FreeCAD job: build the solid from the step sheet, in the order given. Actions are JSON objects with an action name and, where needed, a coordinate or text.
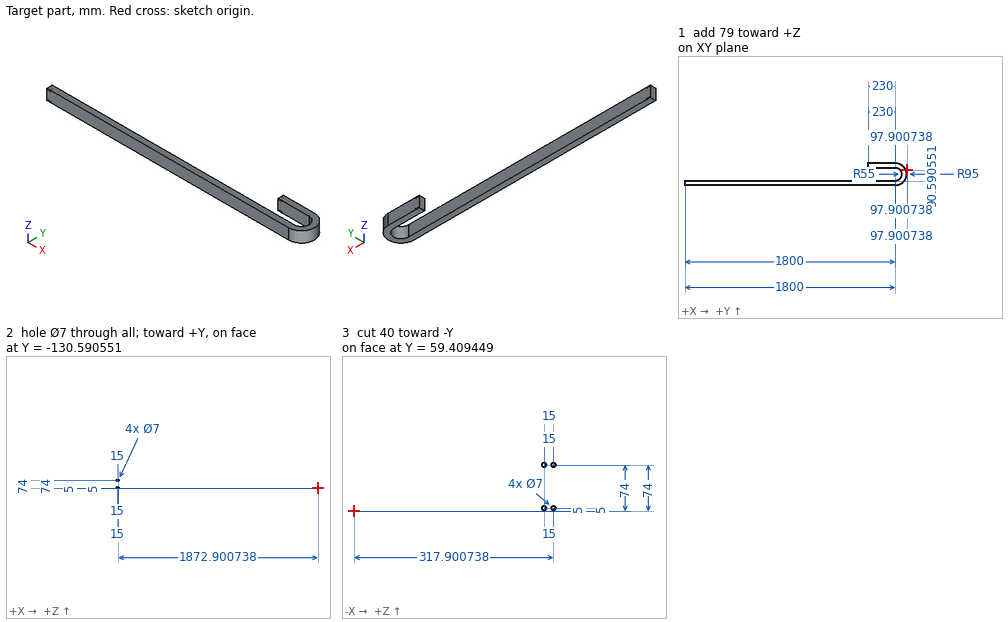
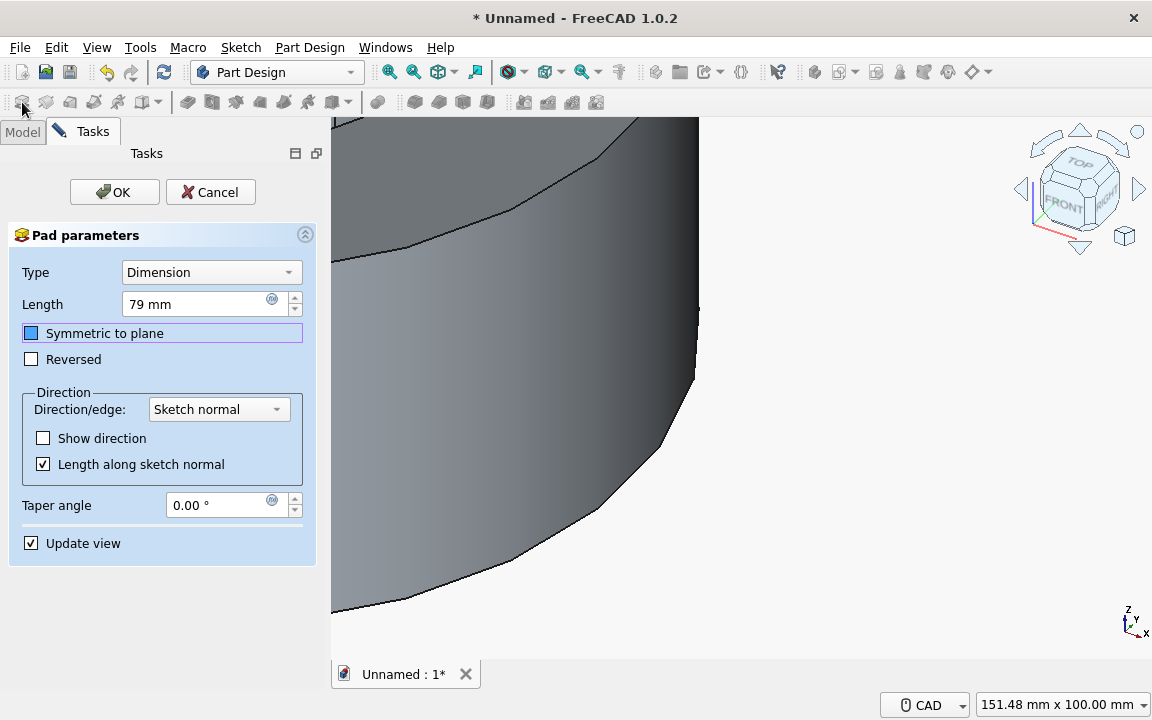
{"action": "left_click", "coordinate": [115, 192]}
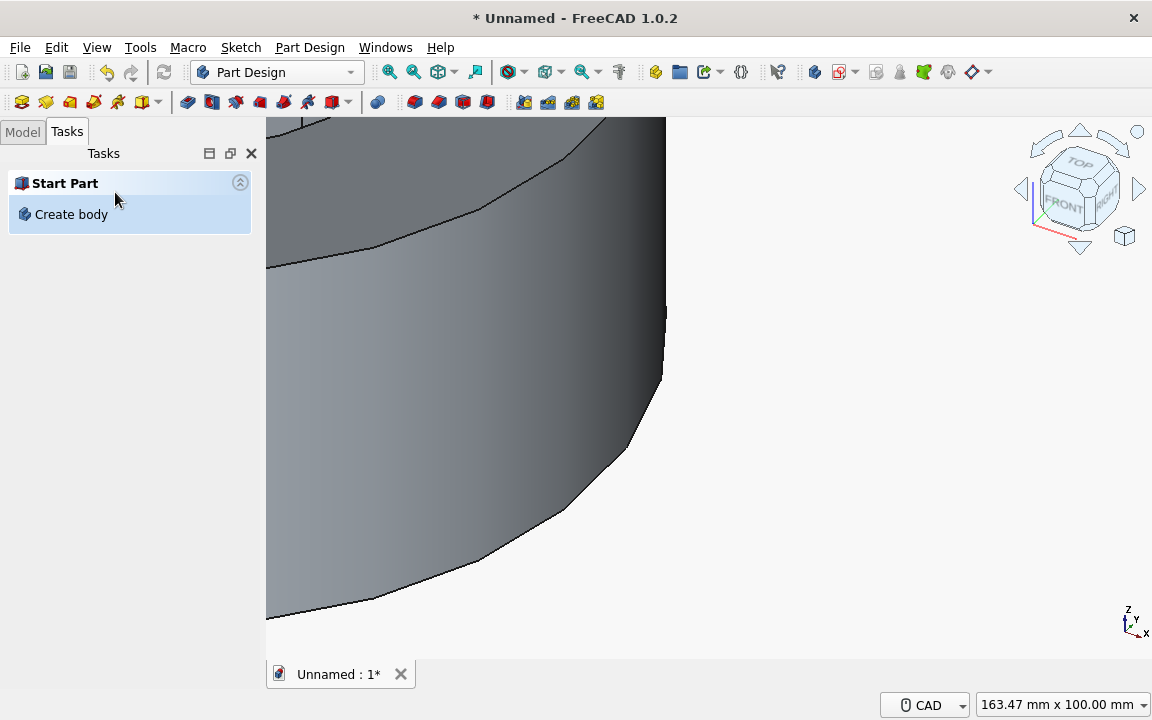
{"action": "left_click", "coordinate": [390, 72]}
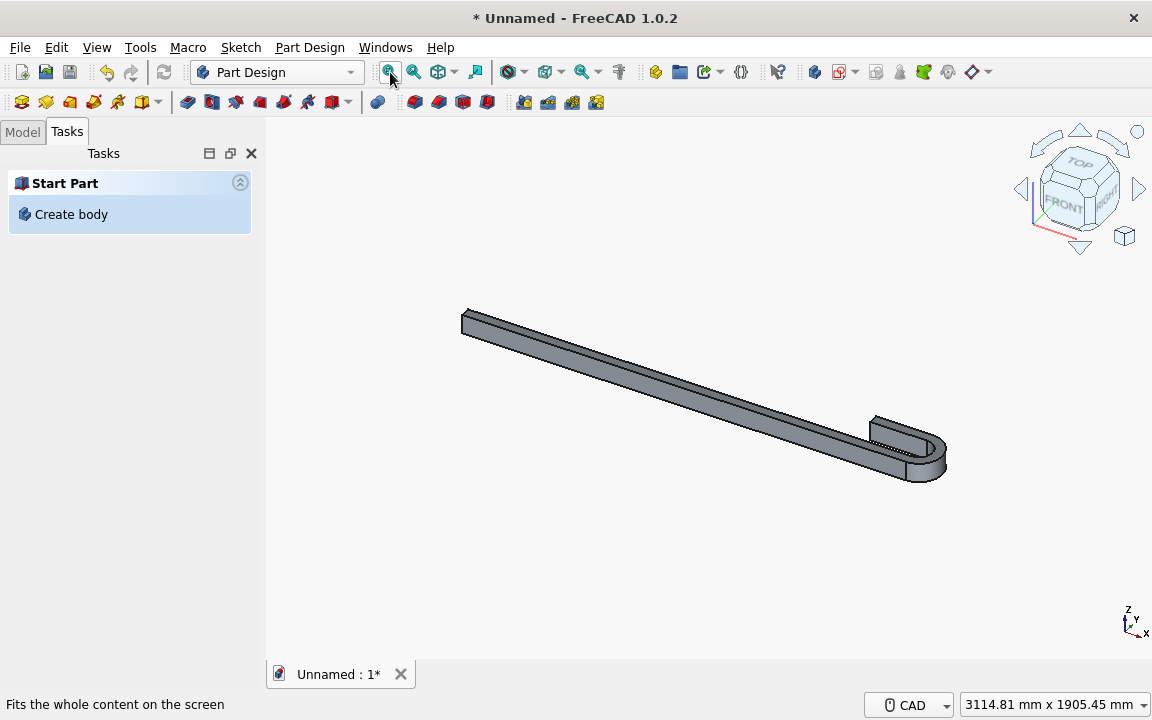
{"action": "left_click", "coordinate": [874, 460]}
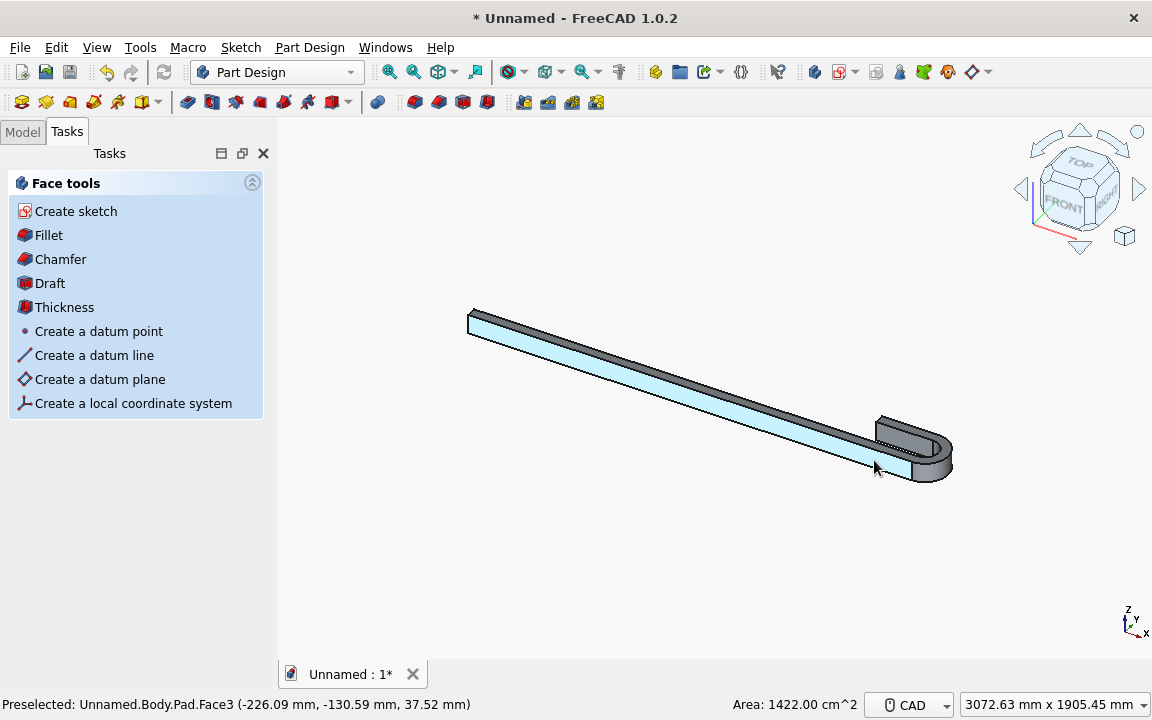
{"action": "left_click", "coordinate": [840, 72]}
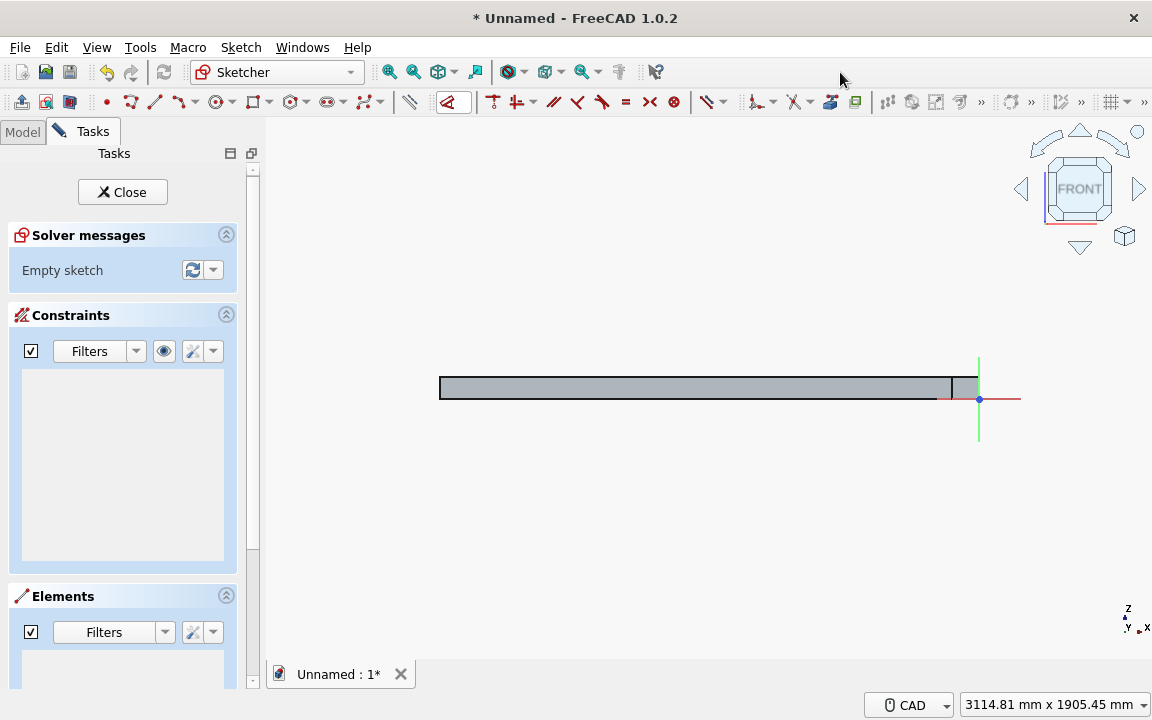
{"action": "scroll", "coordinate": [432, 388], "scroll_direction": "up", "scroll_amount": 14}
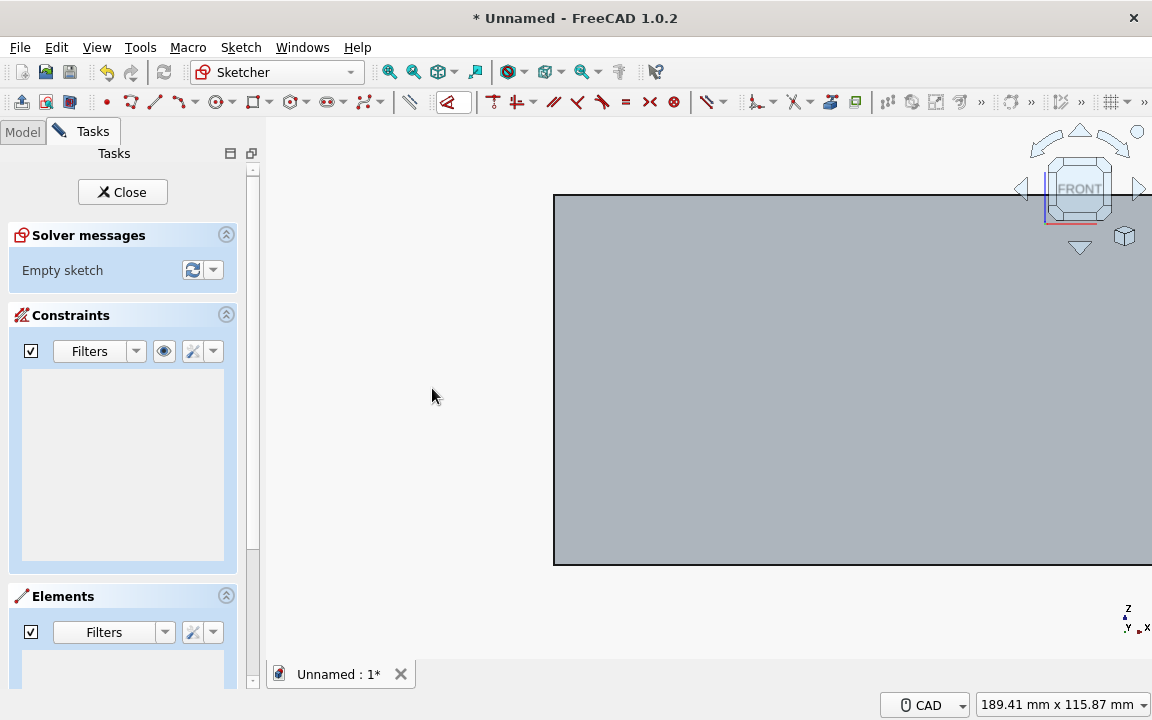
{"action": "key", "text": "g c"}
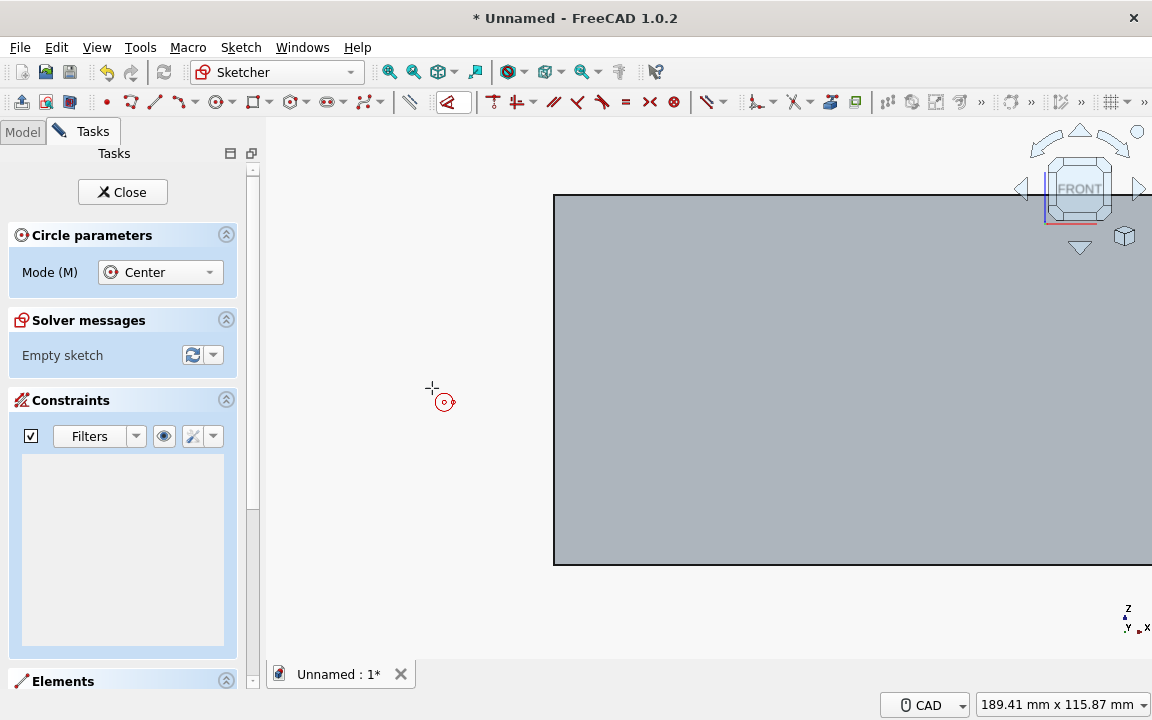
{"action": "scroll", "coordinate": [671, 542], "scroll_direction": "up", "scroll_amount": 2}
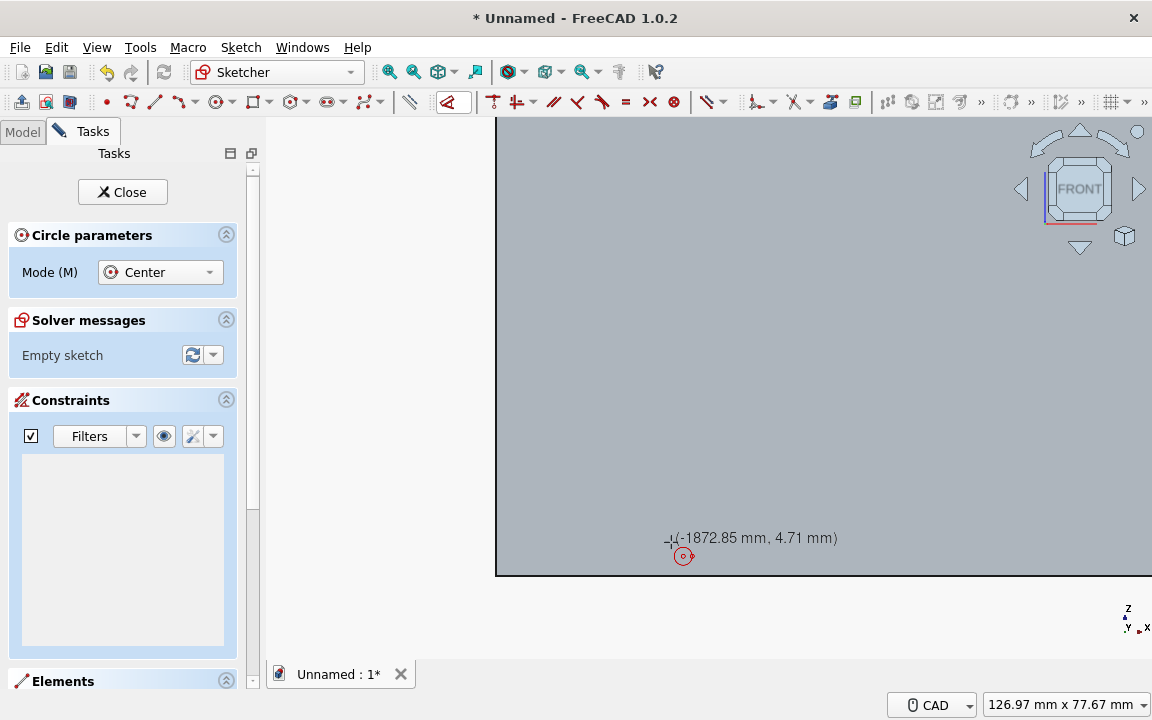
{"action": "left_click", "coordinate": [670, 541]}
{"action": "left_click", "coordinate": [688, 524]}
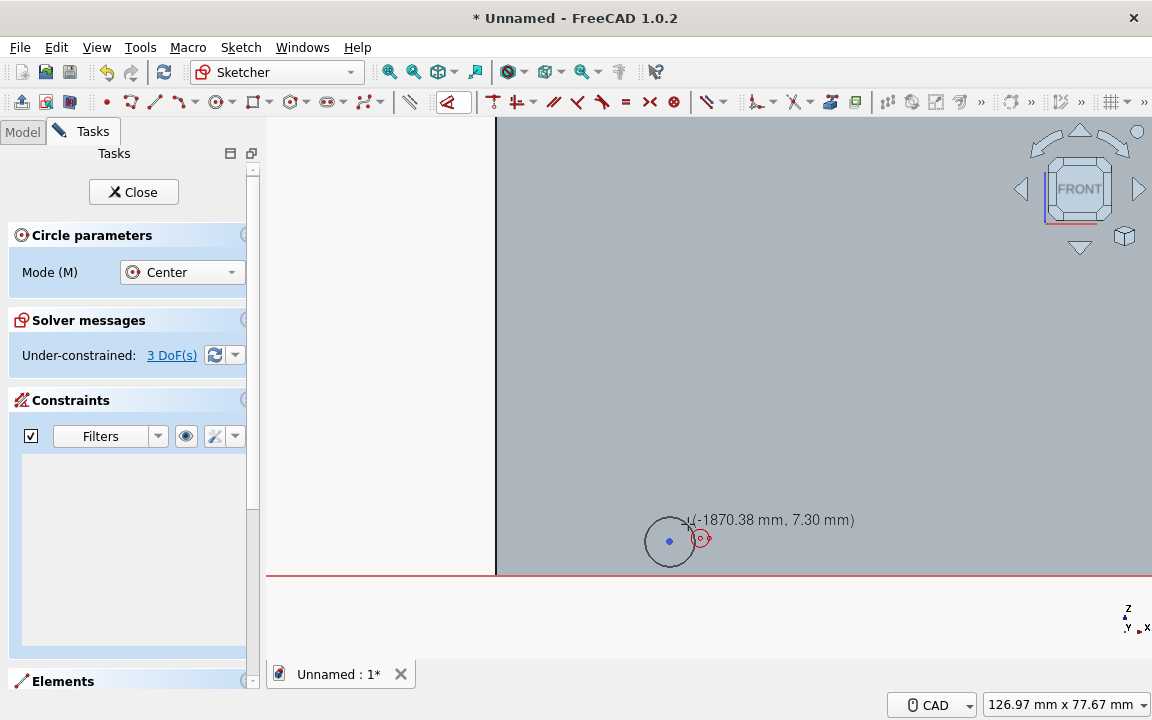
{"action": "left_click", "coordinate": [566, 541]}
{"action": "left_click", "coordinate": [583, 524]}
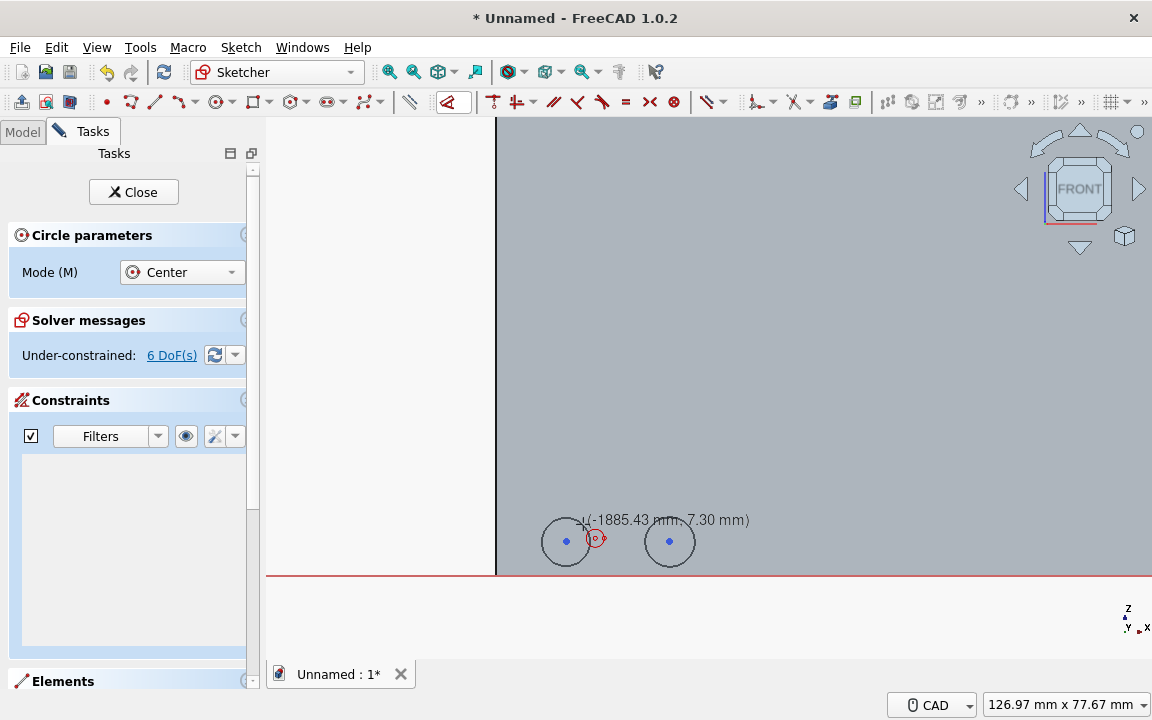
{"action": "scroll", "coordinate": [686, 566], "scroll_direction": "down", "scroll_amount": 2}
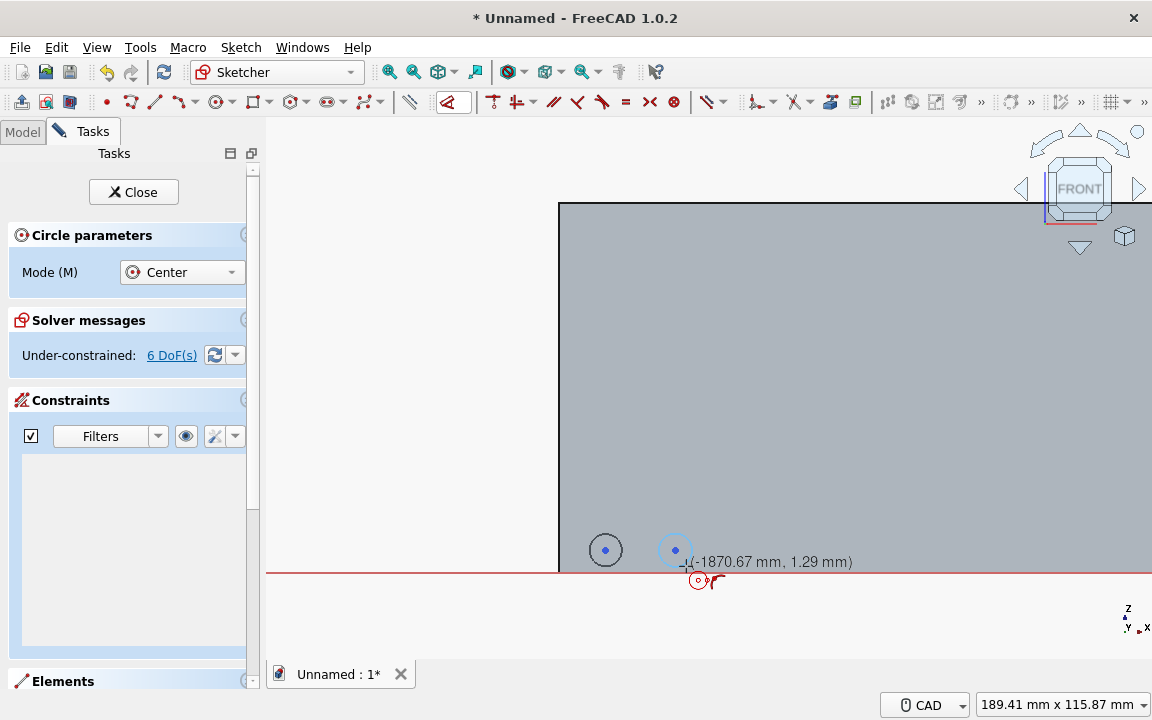
{"action": "scroll", "coordinate": [676, 227], "scroll_direction": "up", "scroll_amount": 2}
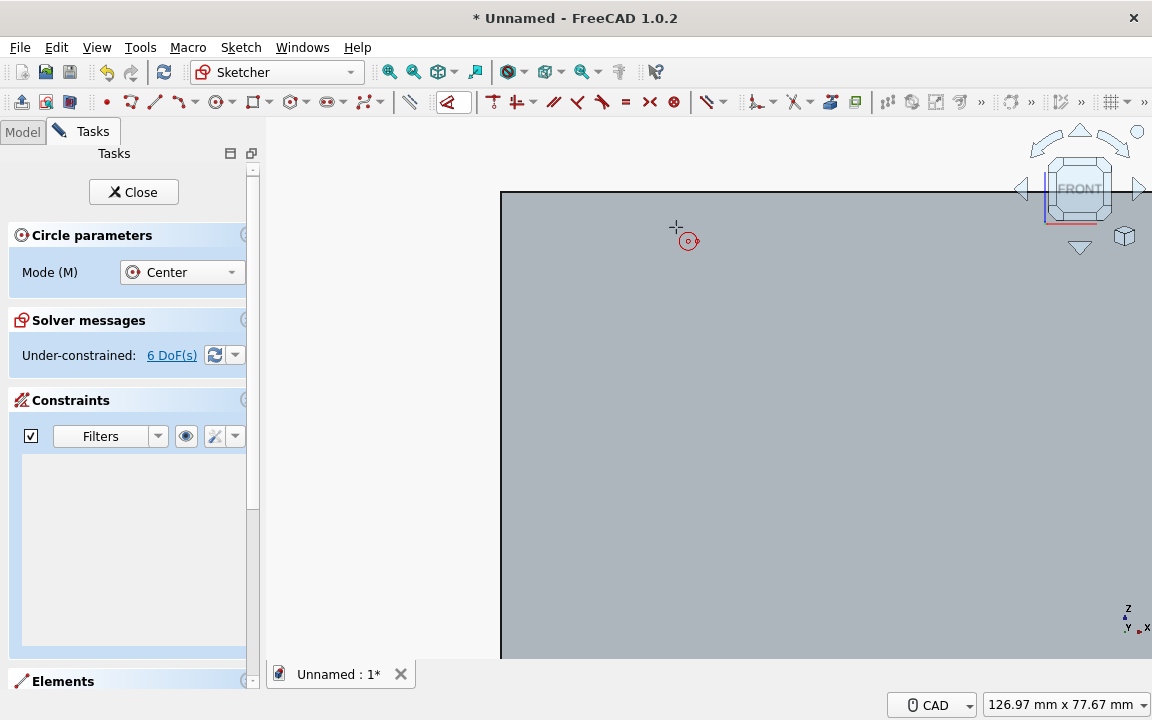
{"action": "left_click", "coordinate": [675, 227]}
{"action": "left_click", "coordinate": [693, 209]}